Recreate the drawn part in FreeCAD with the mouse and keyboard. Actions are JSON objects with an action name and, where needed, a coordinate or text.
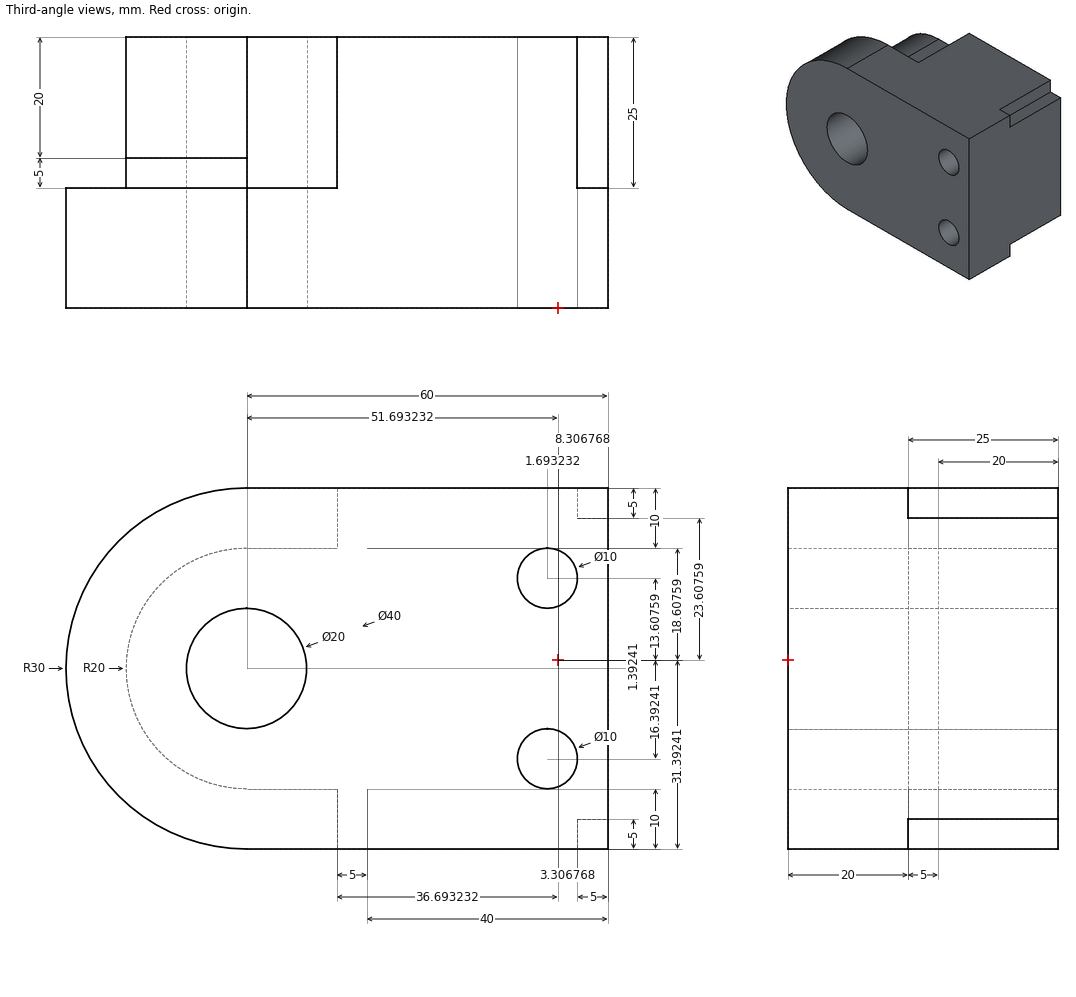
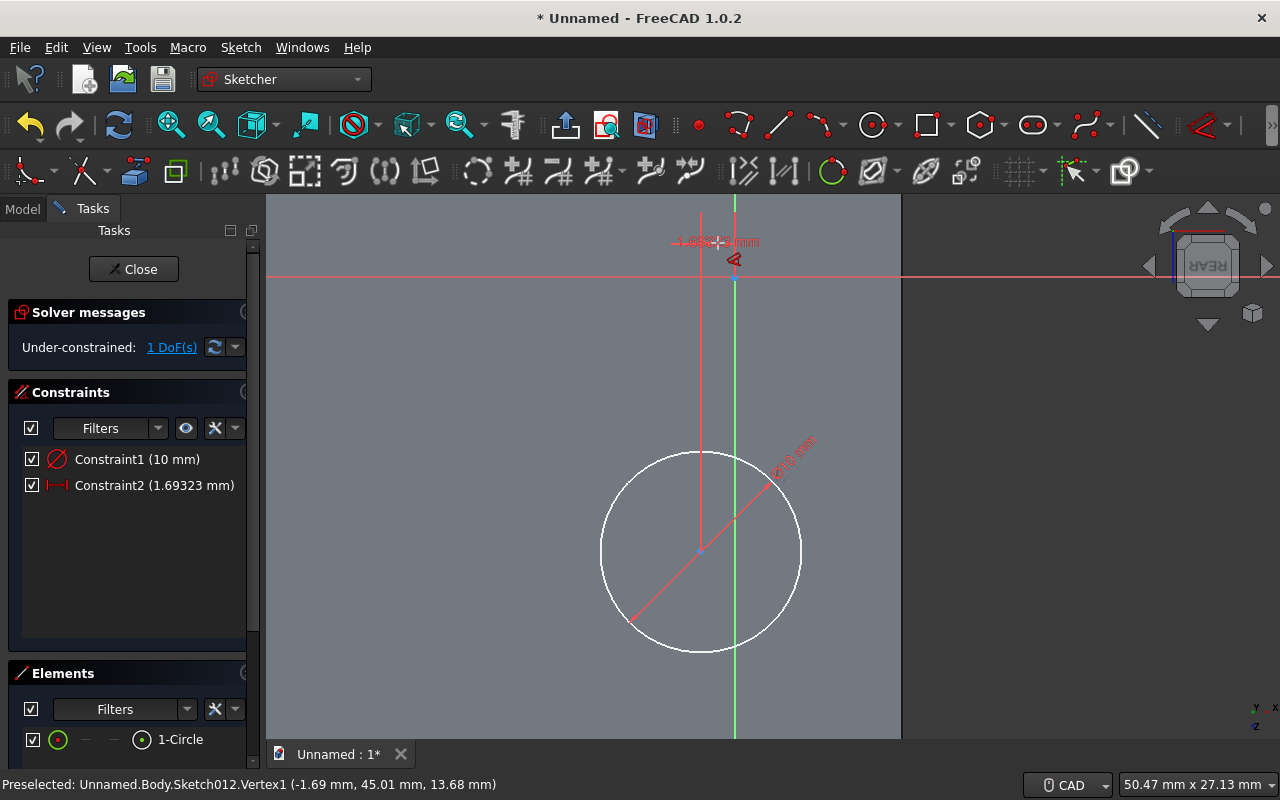
{"action": "left_click", "coordinate": [701, 552]}
{"action": "left_click", "coordinate": [769, 415]}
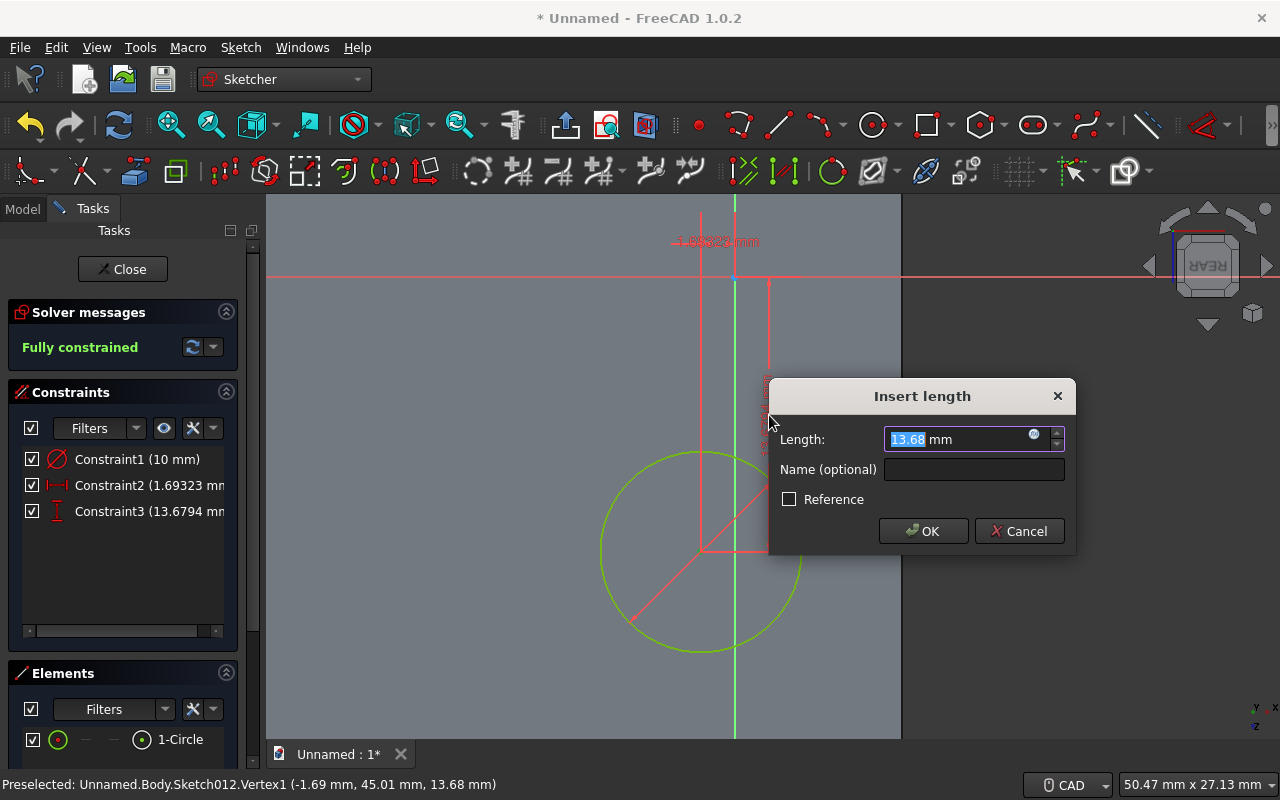
{"action": "type", "text": "13.60759"}
{"action": "key", "text": "Return"}
{"action": "key", "text": "Escape"}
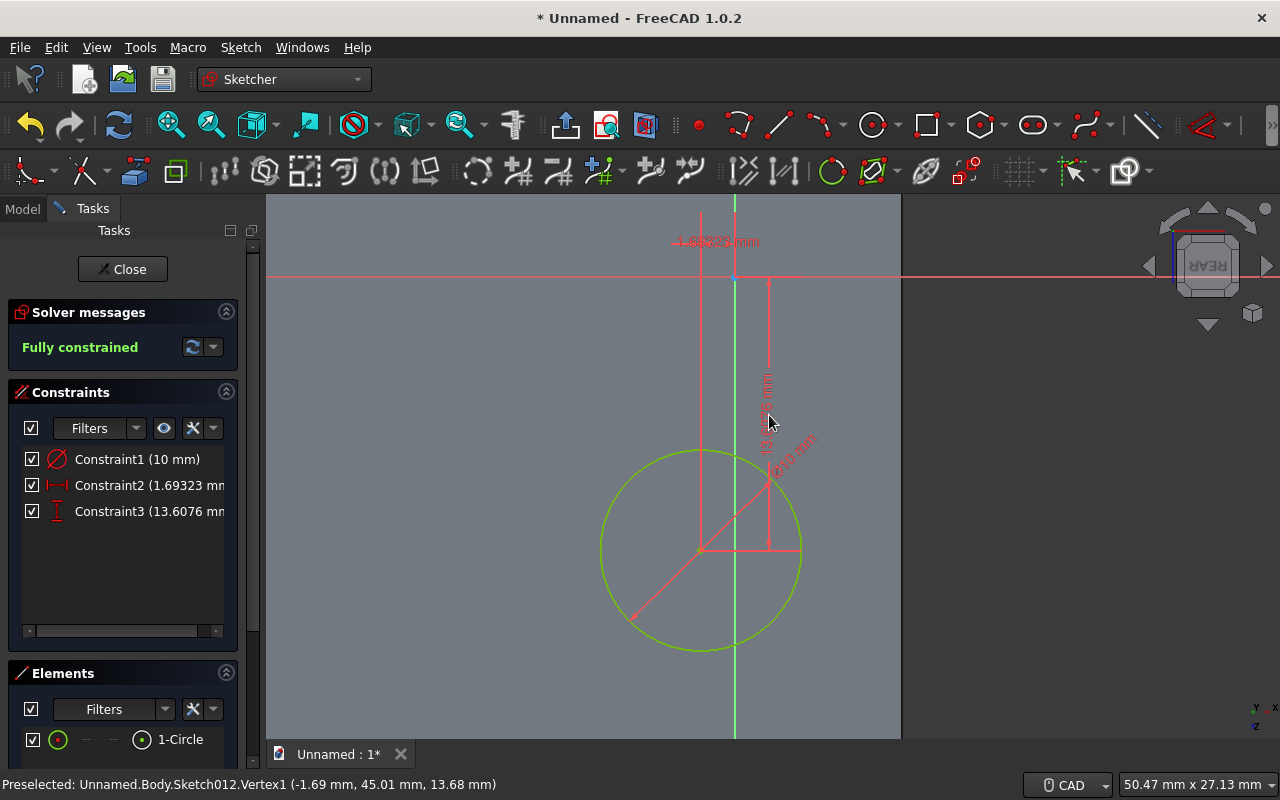
{"action": "left_click", "coordinate": [123, 269]}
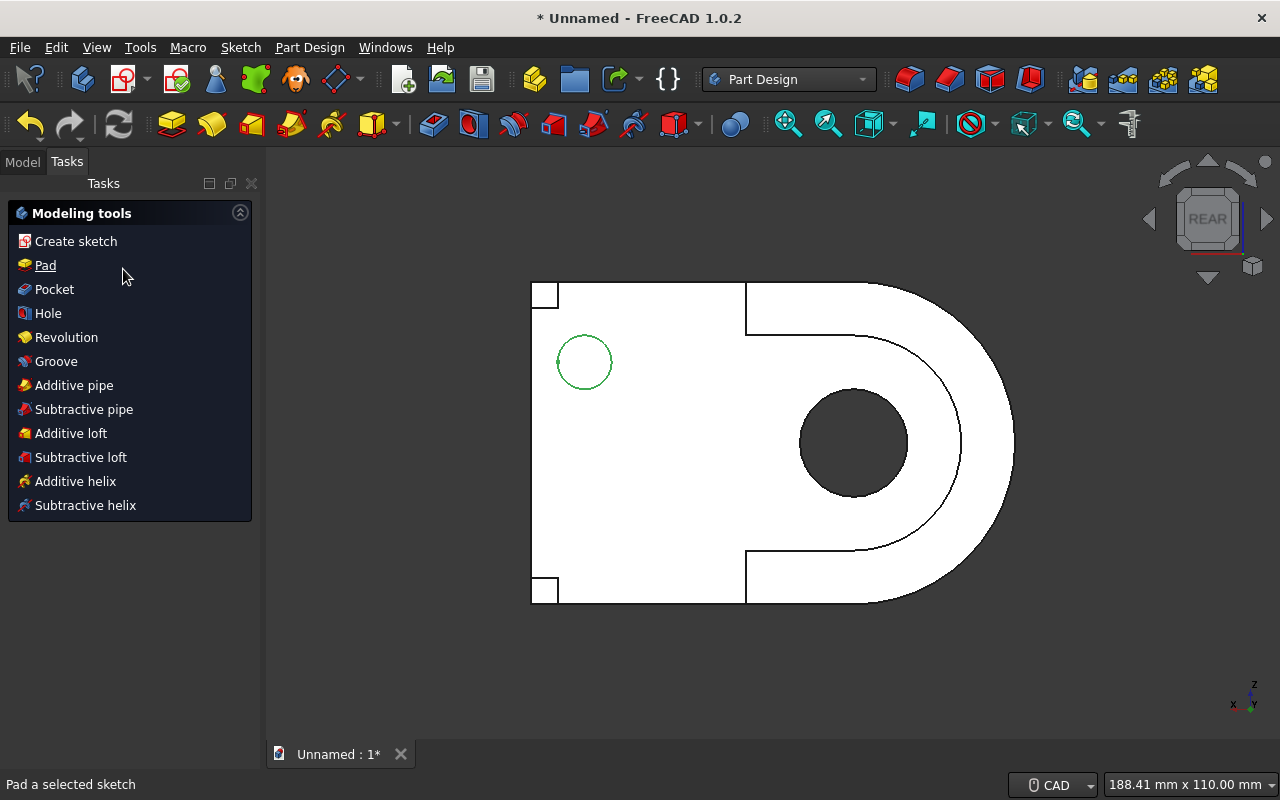
{"action": "left_click", "coordinate": [434, 124]}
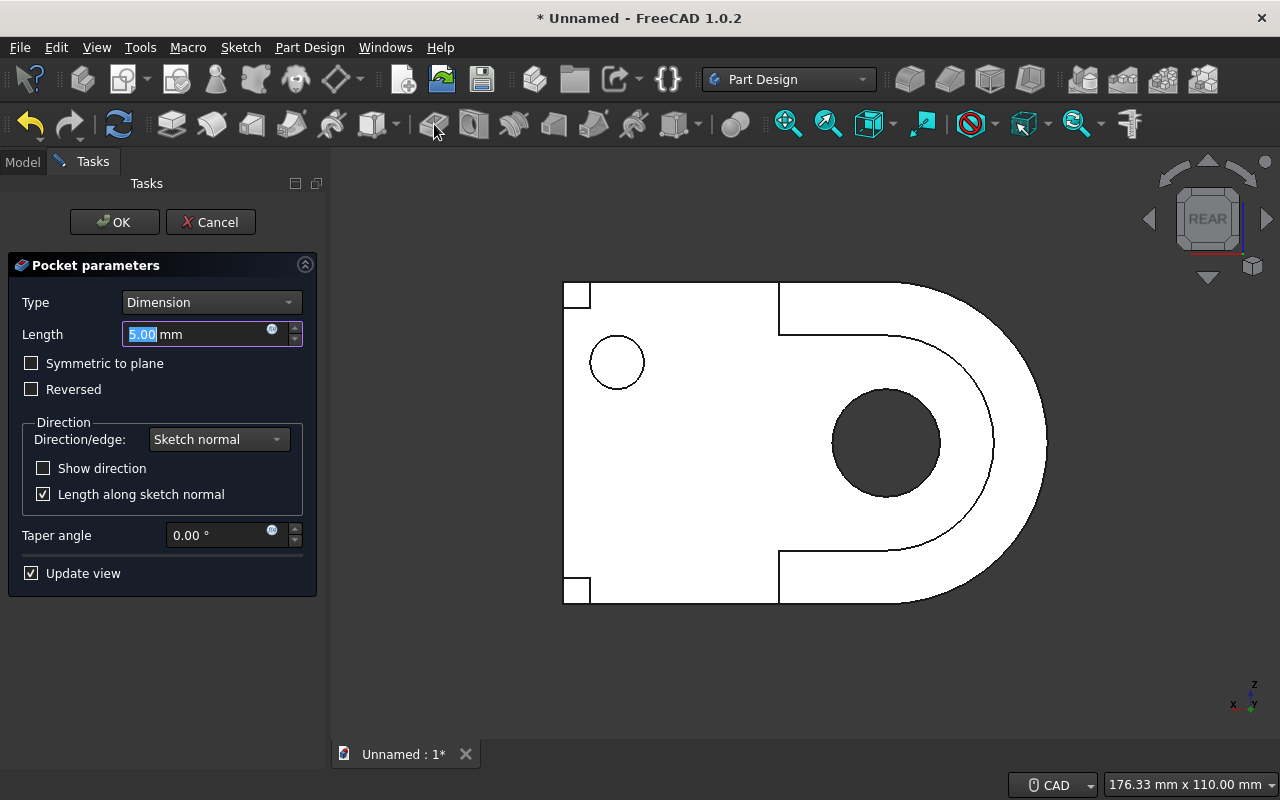
{"action": "left_click", "coordinate": [212, 302]}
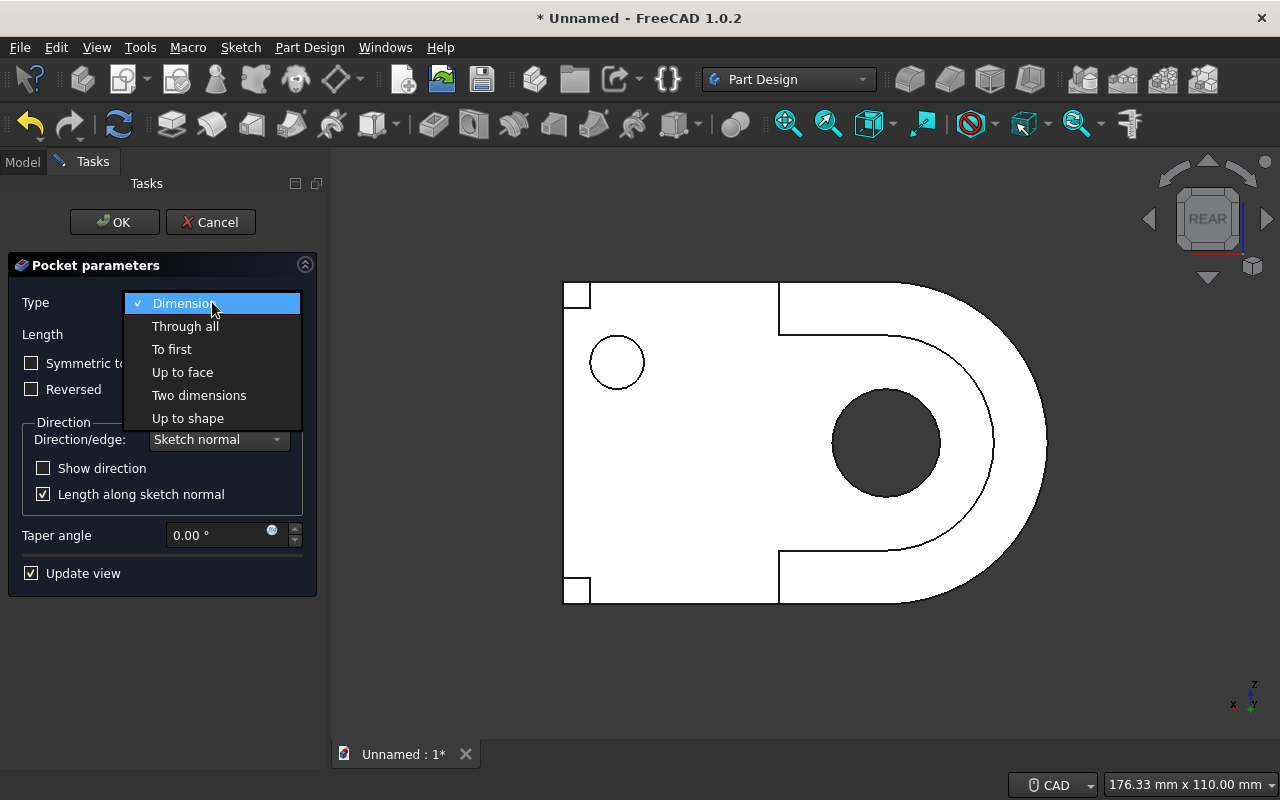
{"action": "left_click", "coordinate": [212, 396]}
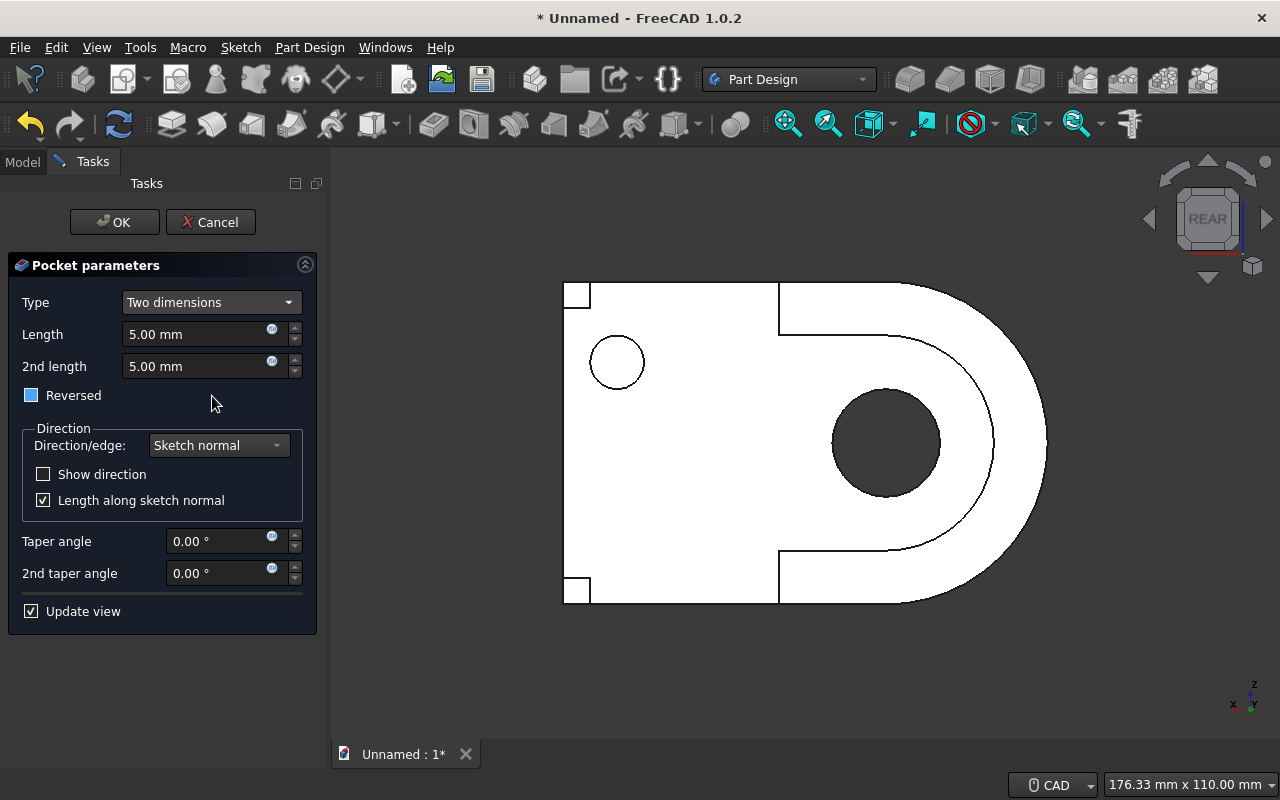
{"action": "triple_click", "coordinate": [204, 334]}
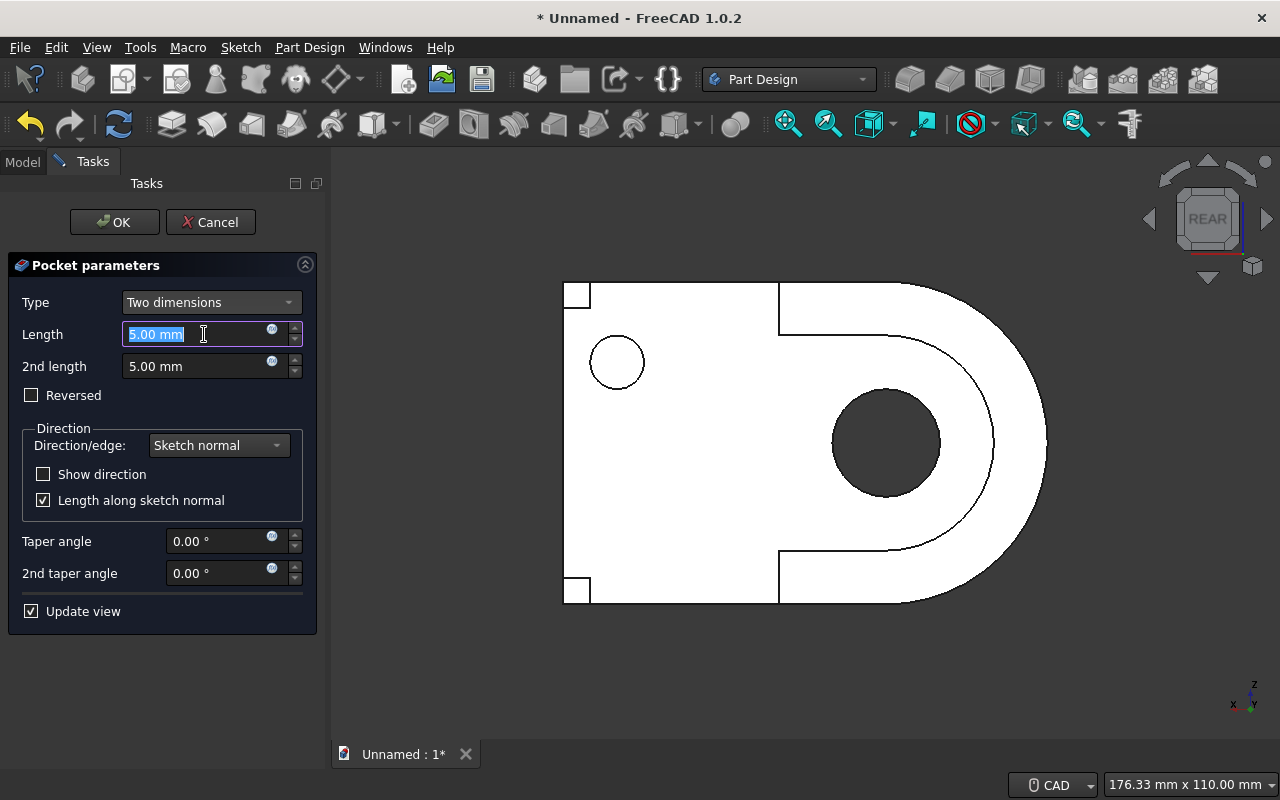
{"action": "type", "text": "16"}
{"action": "key", "text": "Tab"}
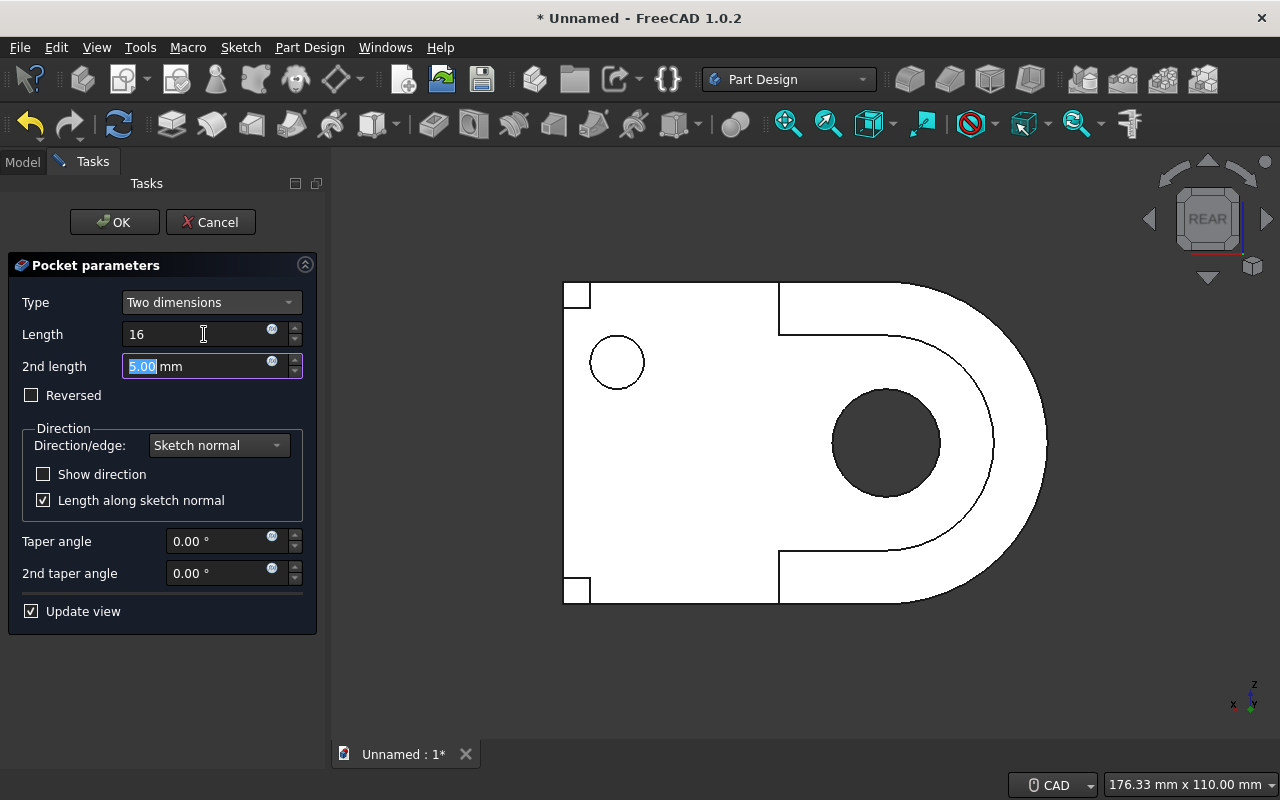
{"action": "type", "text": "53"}
{"action": "key", "text": "Tab"}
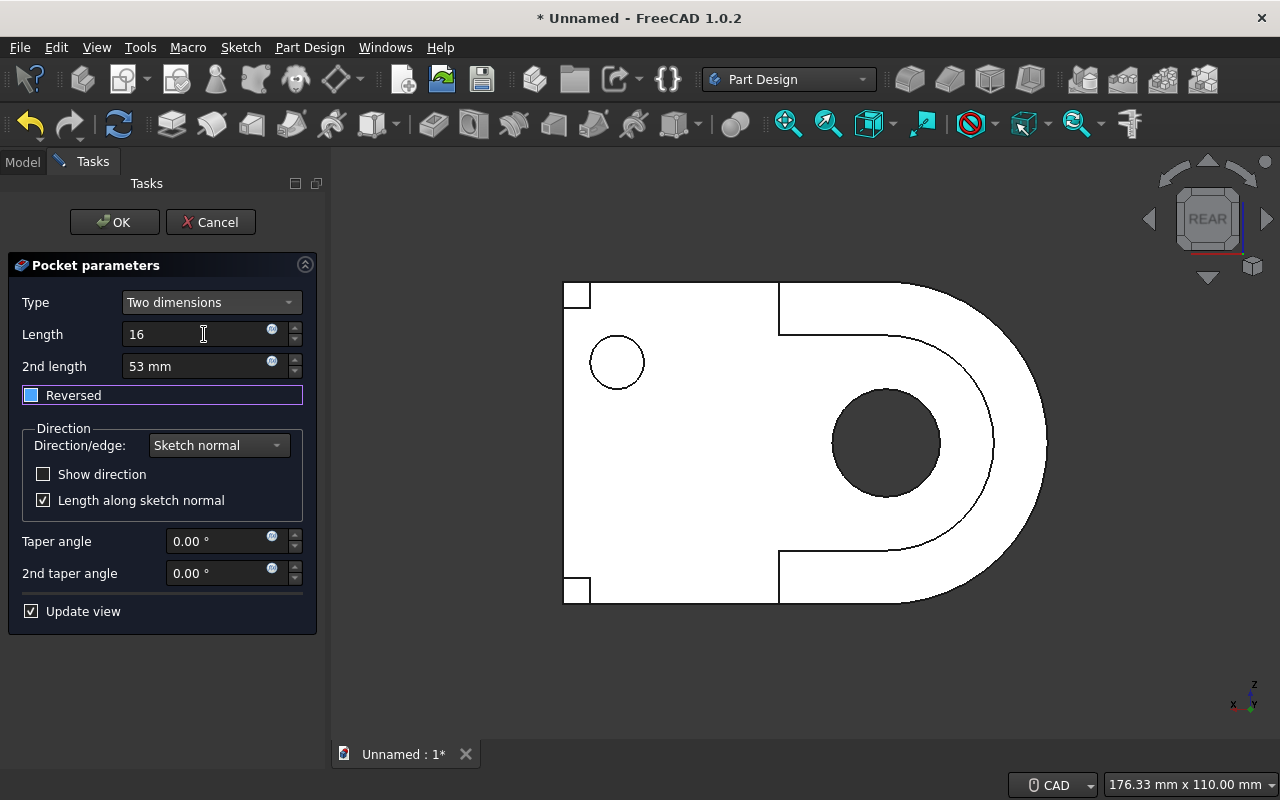
{"action": "left_click", "coordinate": [30, 395]}